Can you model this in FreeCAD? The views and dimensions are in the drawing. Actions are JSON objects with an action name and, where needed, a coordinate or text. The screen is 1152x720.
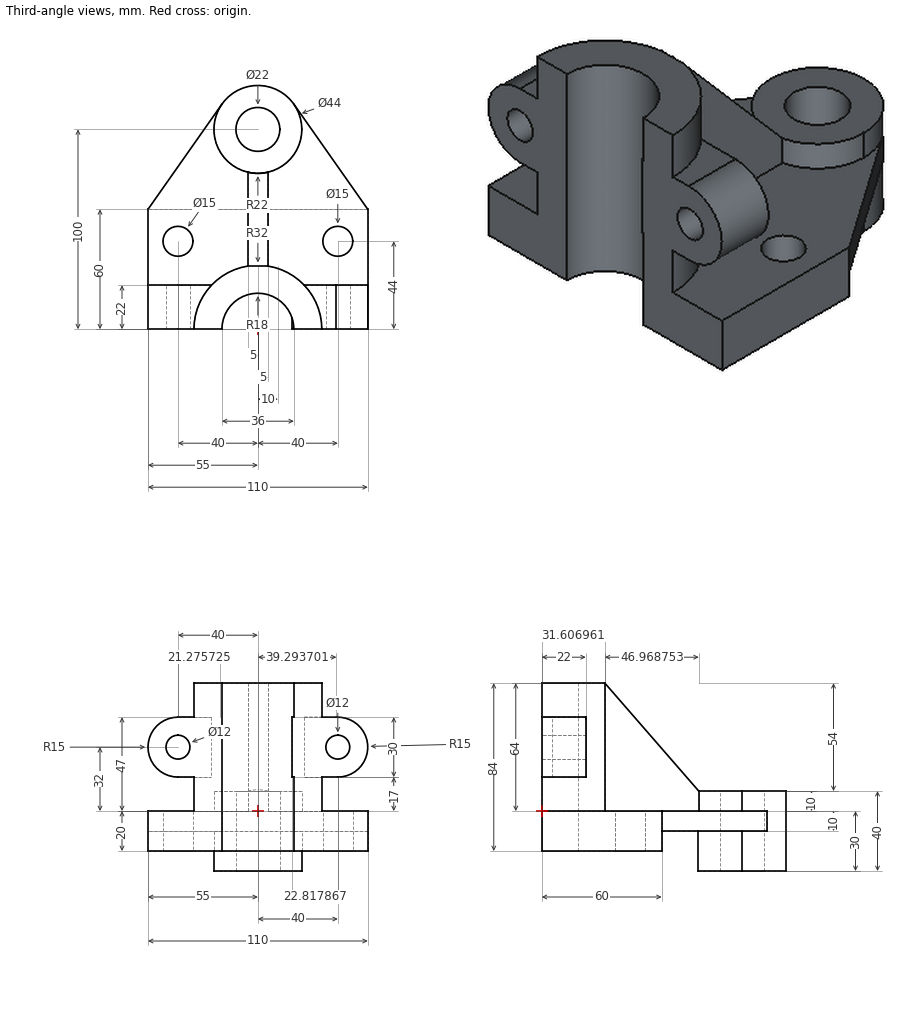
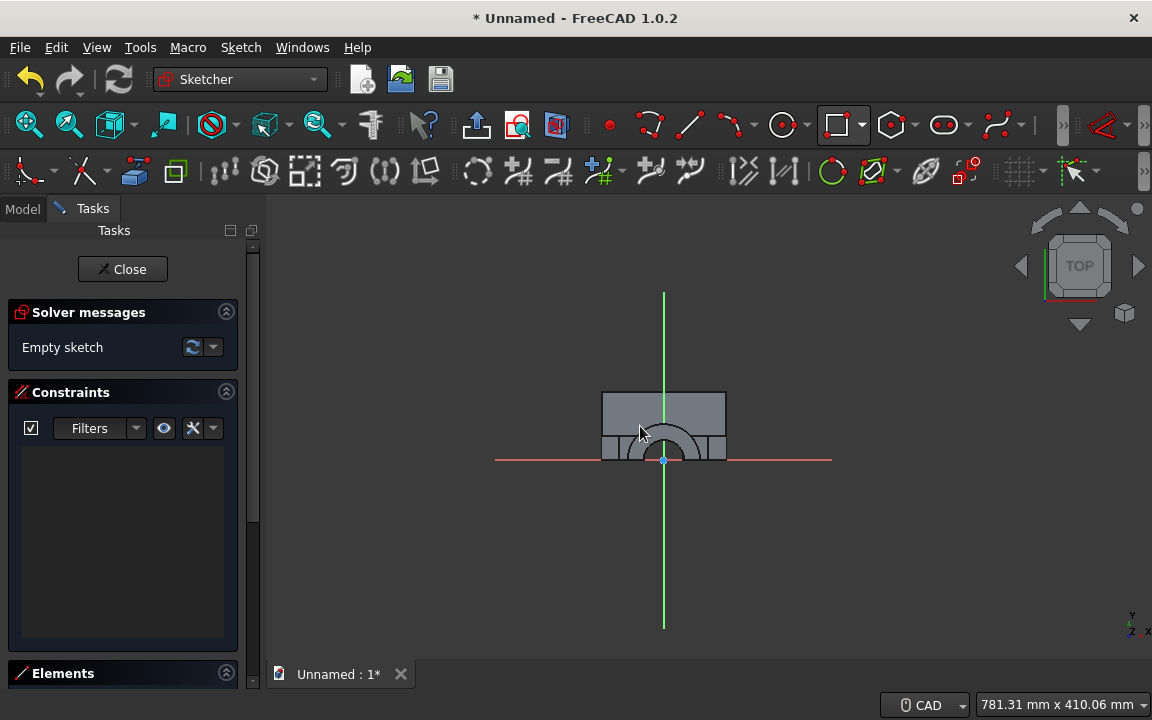
{"action": "scroll", "coordinate": [669, 331], "scroll_direction": "up", "scroll_amount": 9}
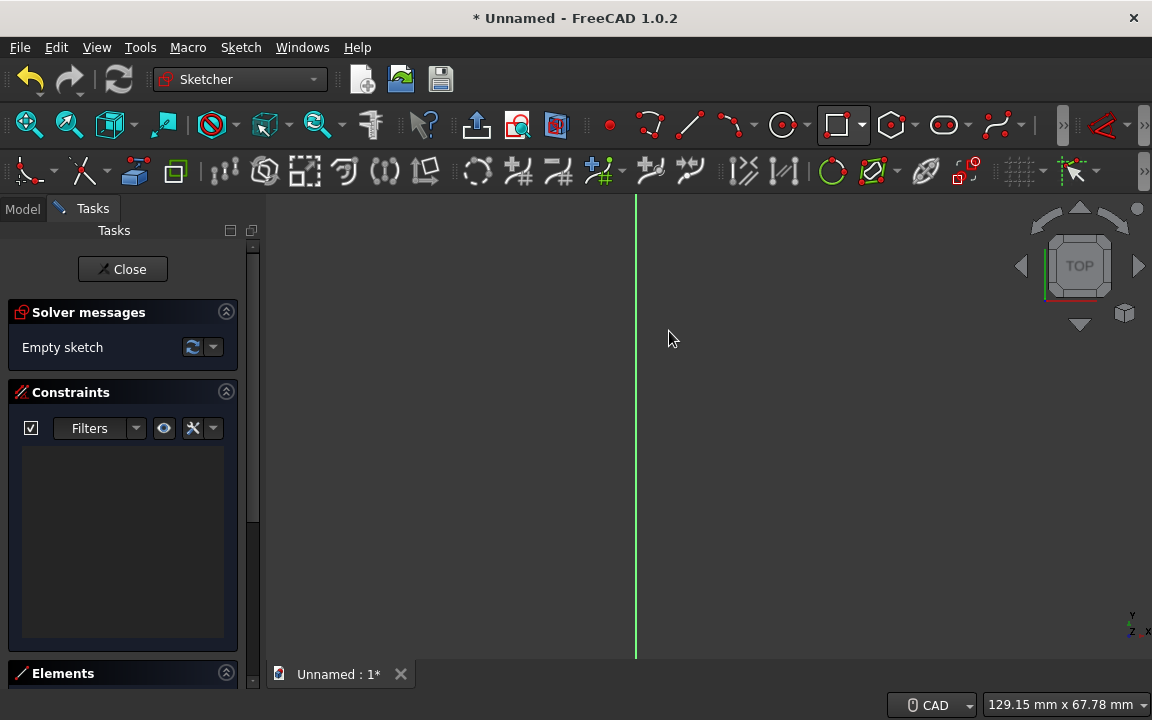
{"action": "left_click", "coordinate": [784, 126]}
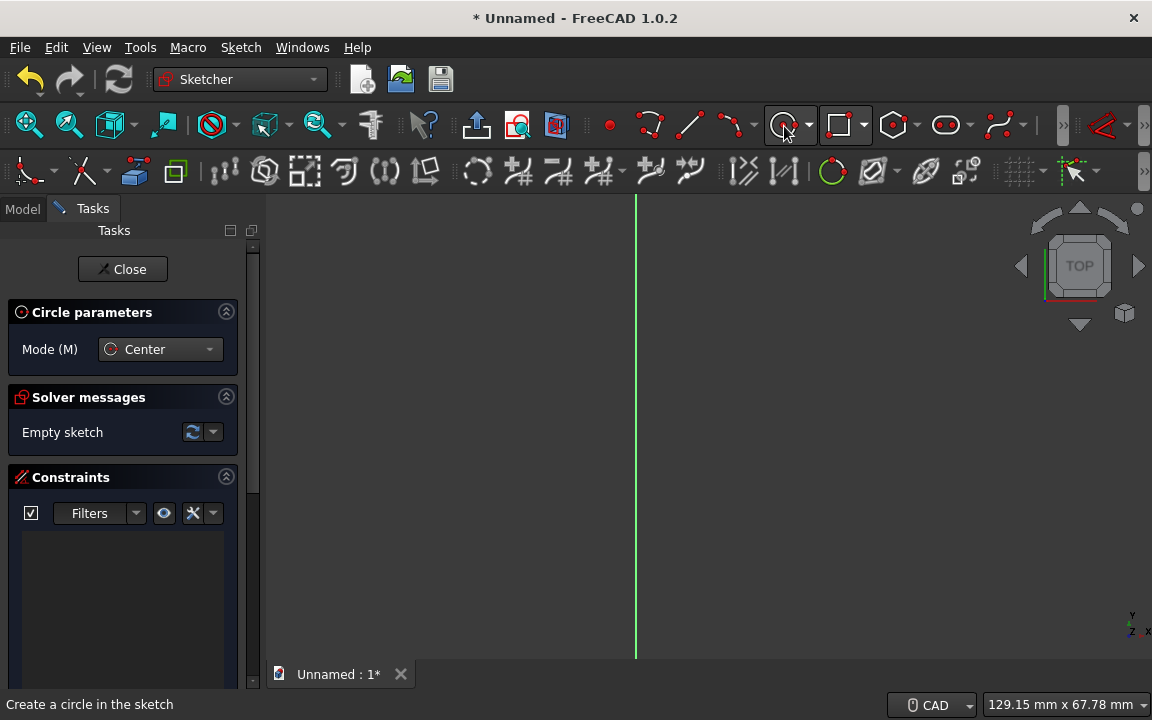
{"action": "left_click", "coordinate": [636, 427]}
{"action": "left_click", "coordinate": [743, 320]}
{"action": "key", "text": "Escape"}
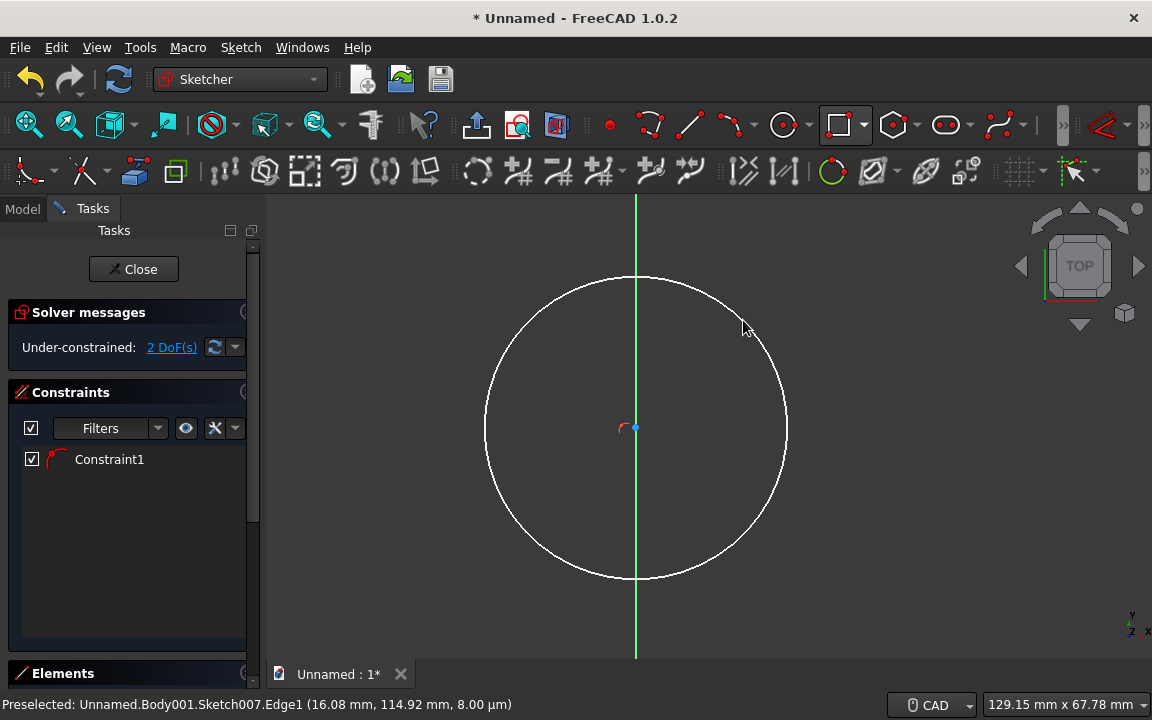
{"action": "left_click", "coordinate": [1102, 126]}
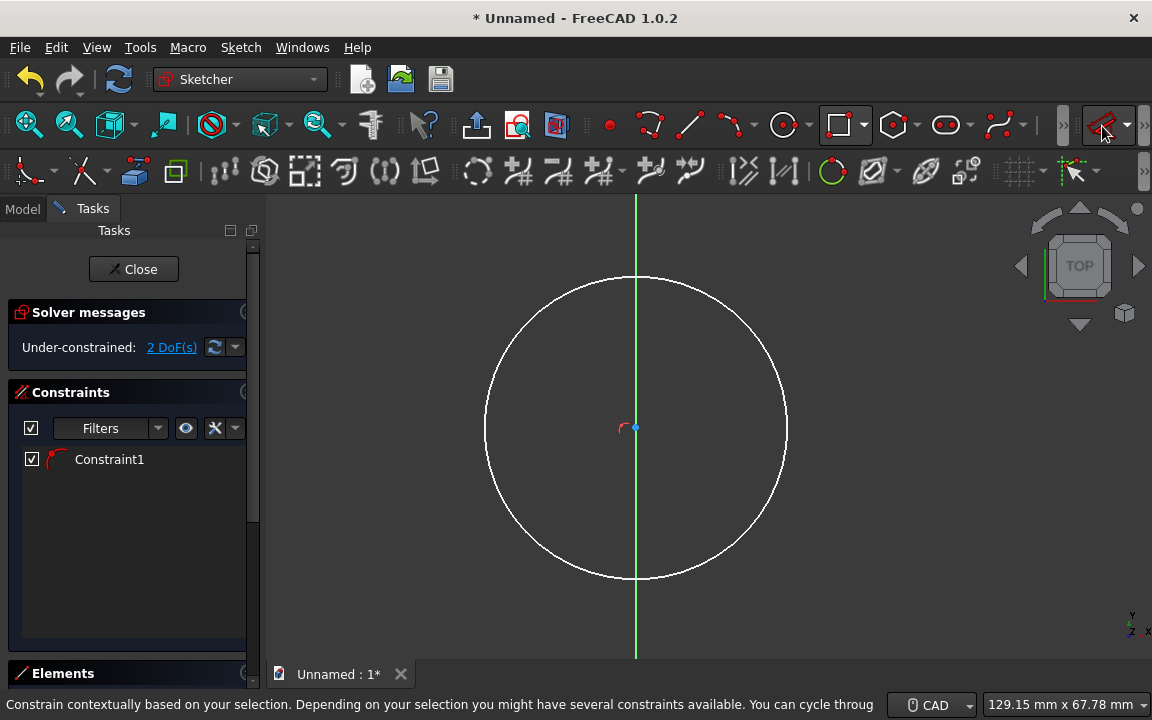
{"action": "left_click", "coordinate": [743, 321]}
{"action": "left_click", "coordinate": [766, 298]}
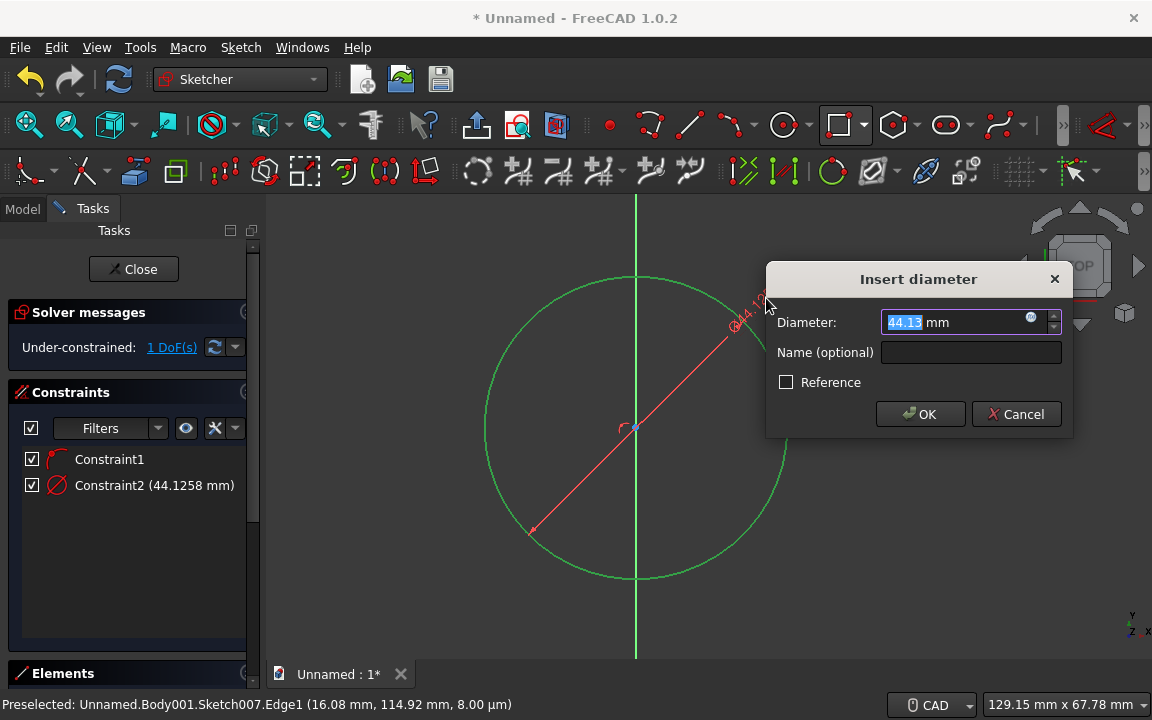
{"action": "type", "text": "44"}
{"action": "key", "text": "Return"}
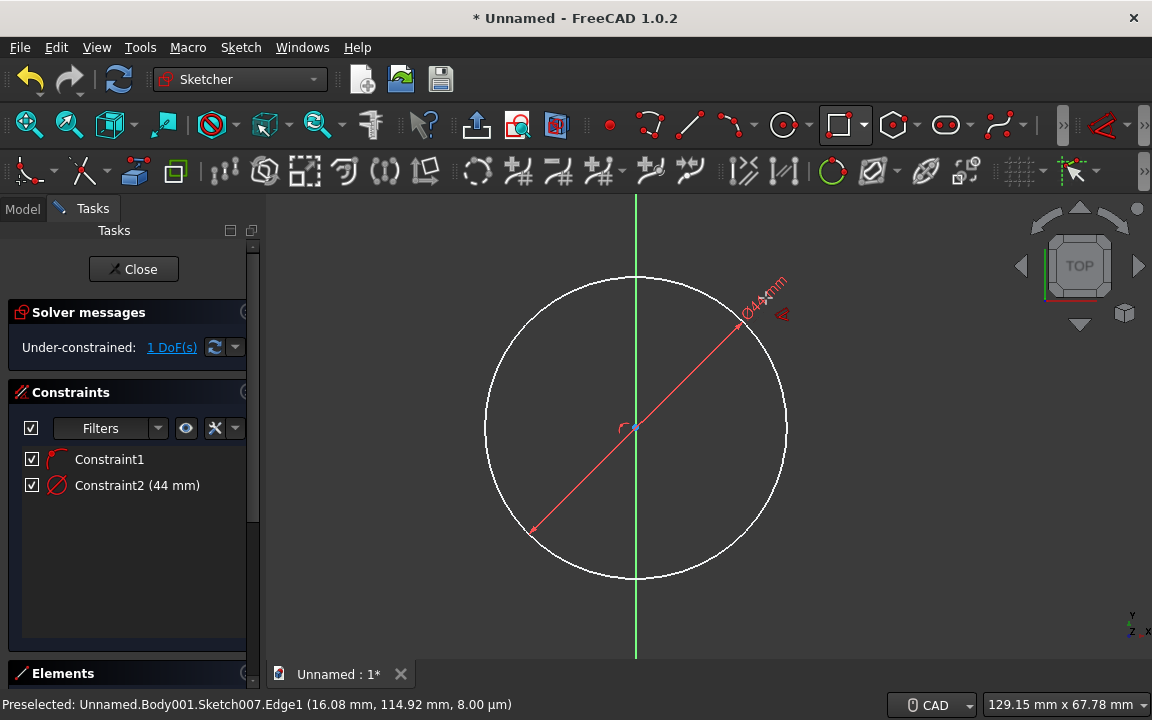
{"action": "left_click", "coordinate": [636, 428]}
{"action": "left_click", "coordinate": [670, 529]}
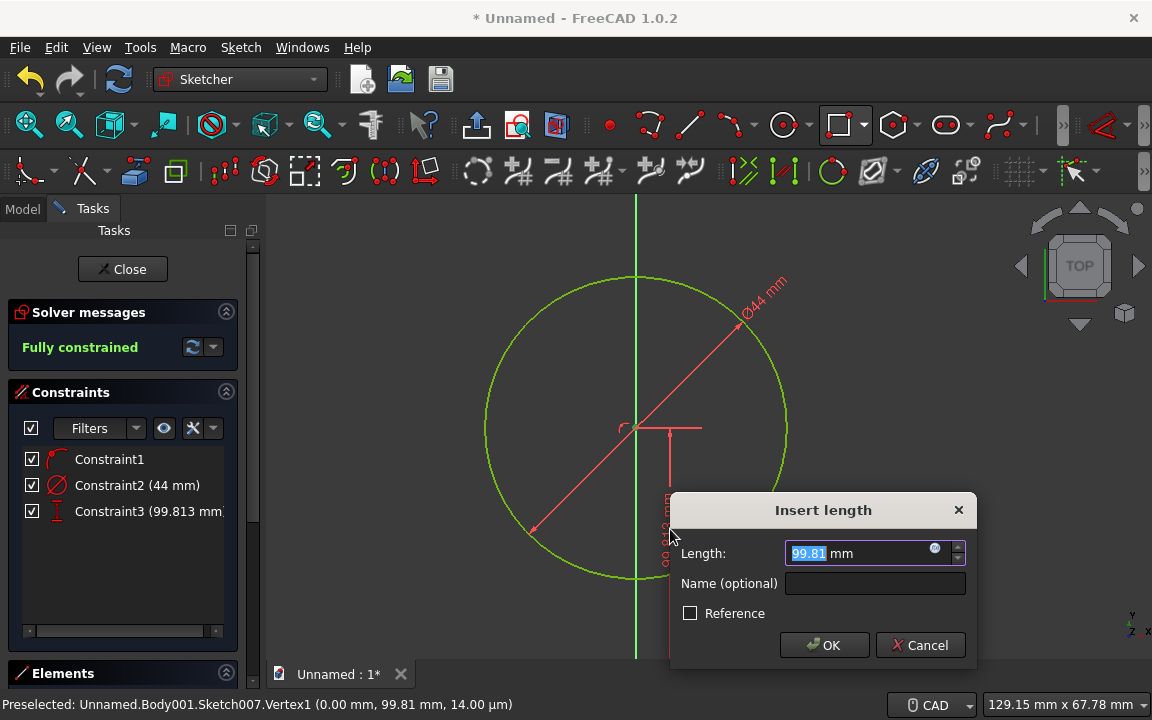
{"action": "type", "text": "100"}
{"action": "key", "text": "Return"}
{"action": "key", "text": "Escape"}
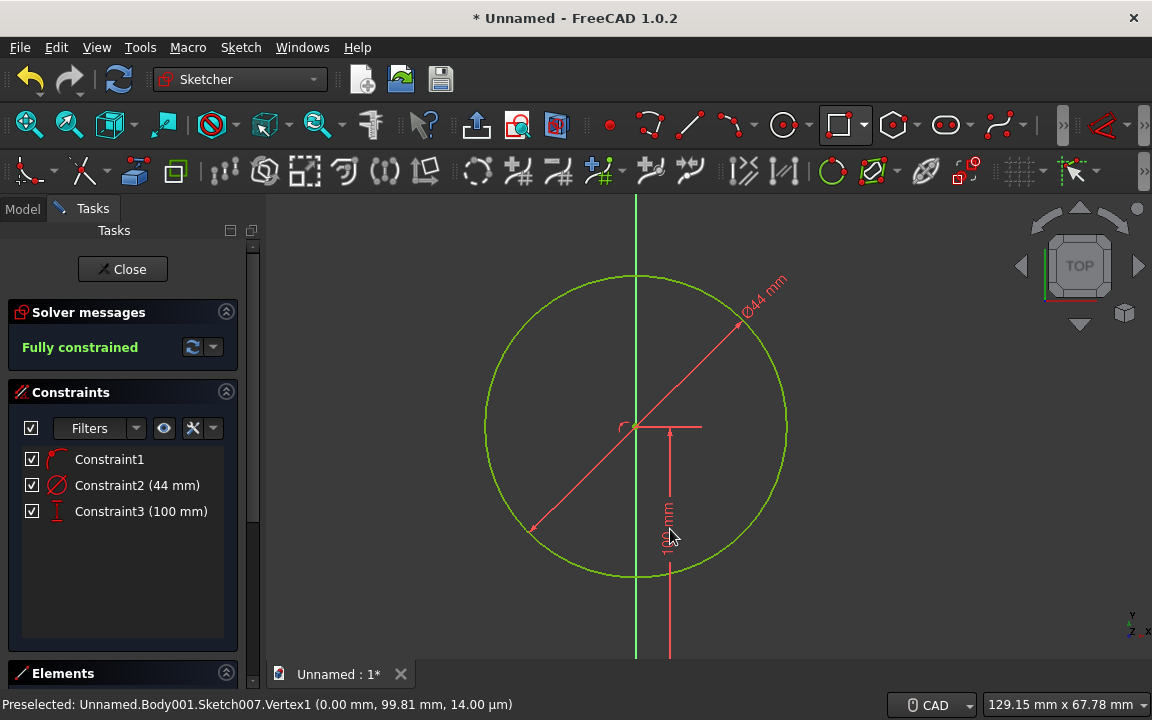
{"action": "left_click", "coordinate": [123, 269]}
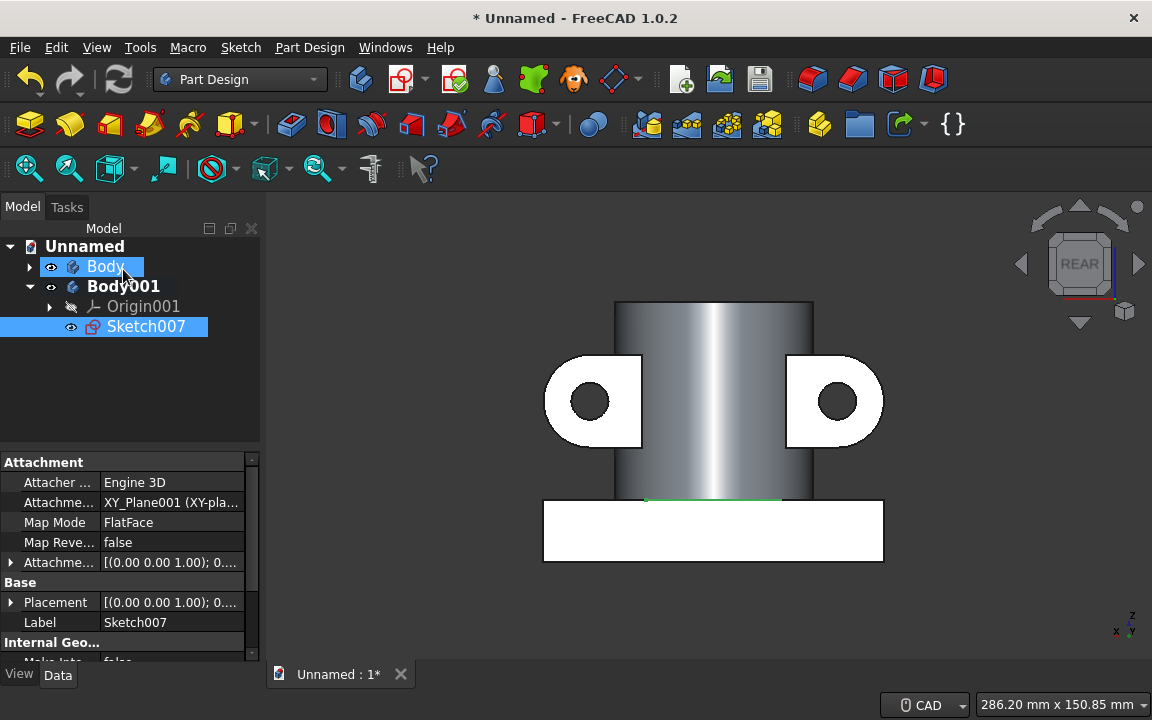
{"action": "left_click", "coordinate": [30, 124]}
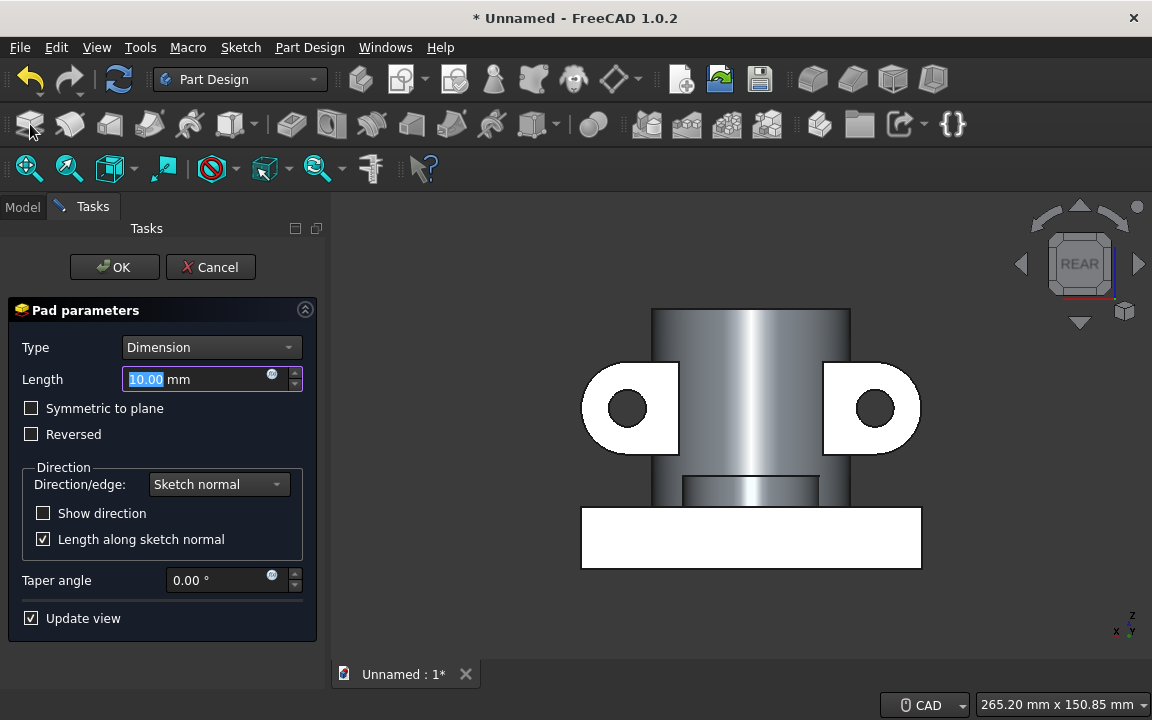
{"action": "left_click", "coordinate": [212, 348]}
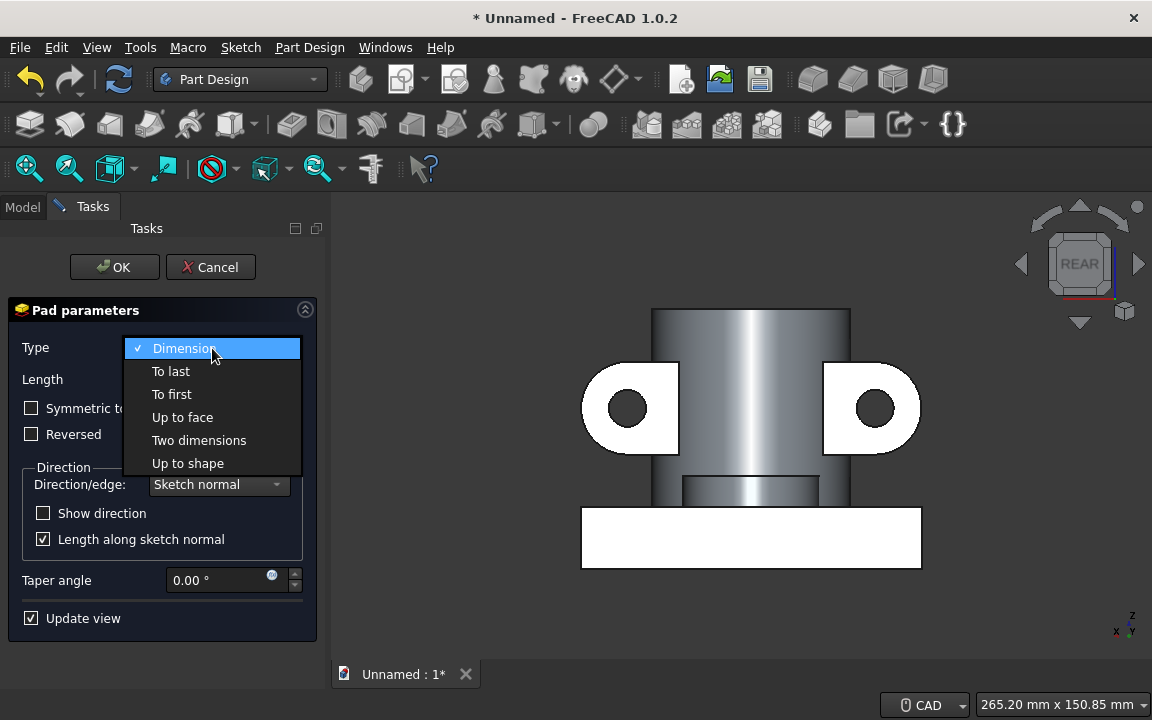
{"action": "left_click", "coordinate": [212, 440]}